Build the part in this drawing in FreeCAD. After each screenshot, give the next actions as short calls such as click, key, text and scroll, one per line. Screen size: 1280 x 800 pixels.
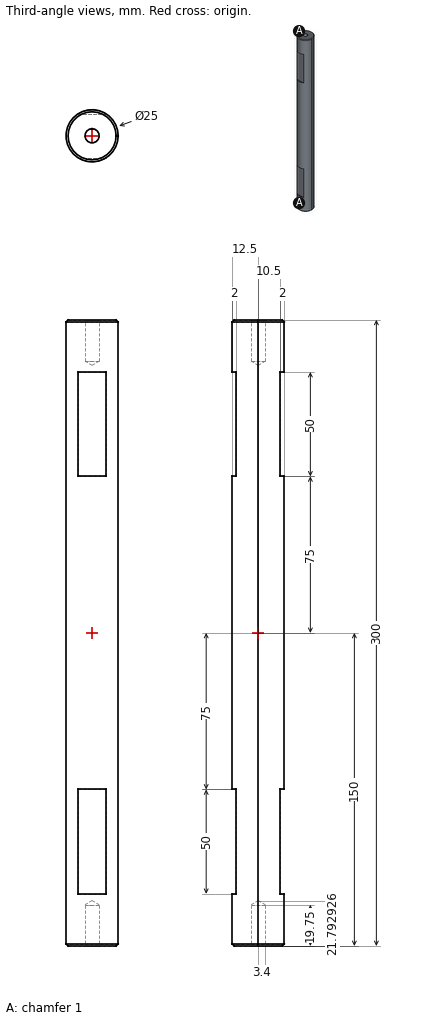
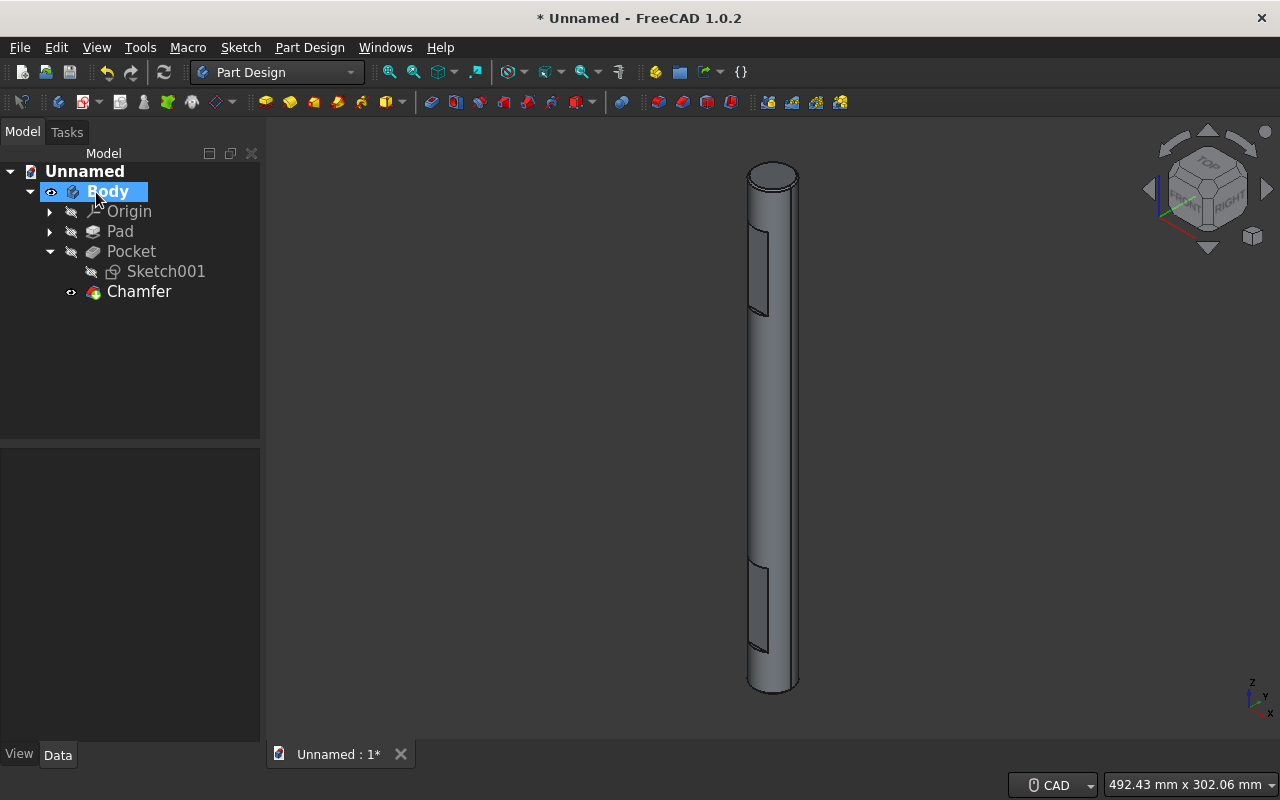
click(84, 102)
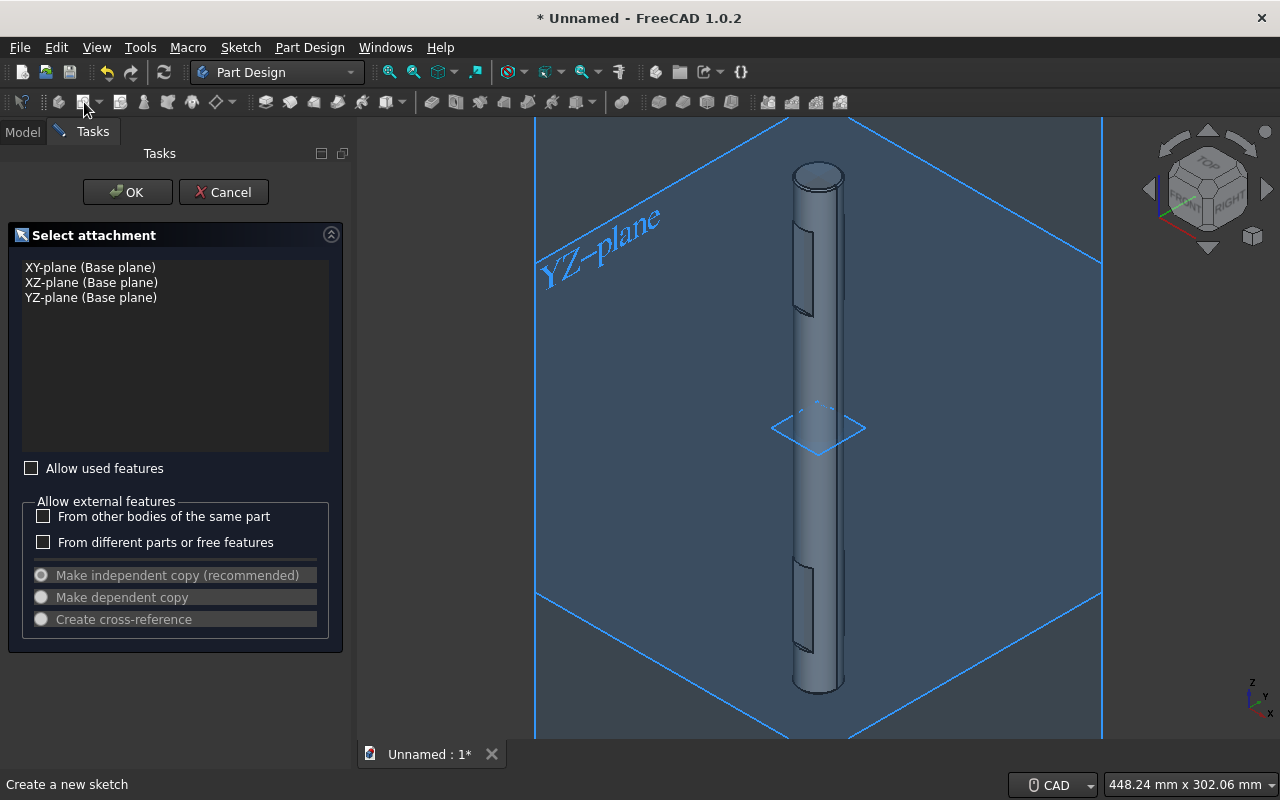
click(82, 298)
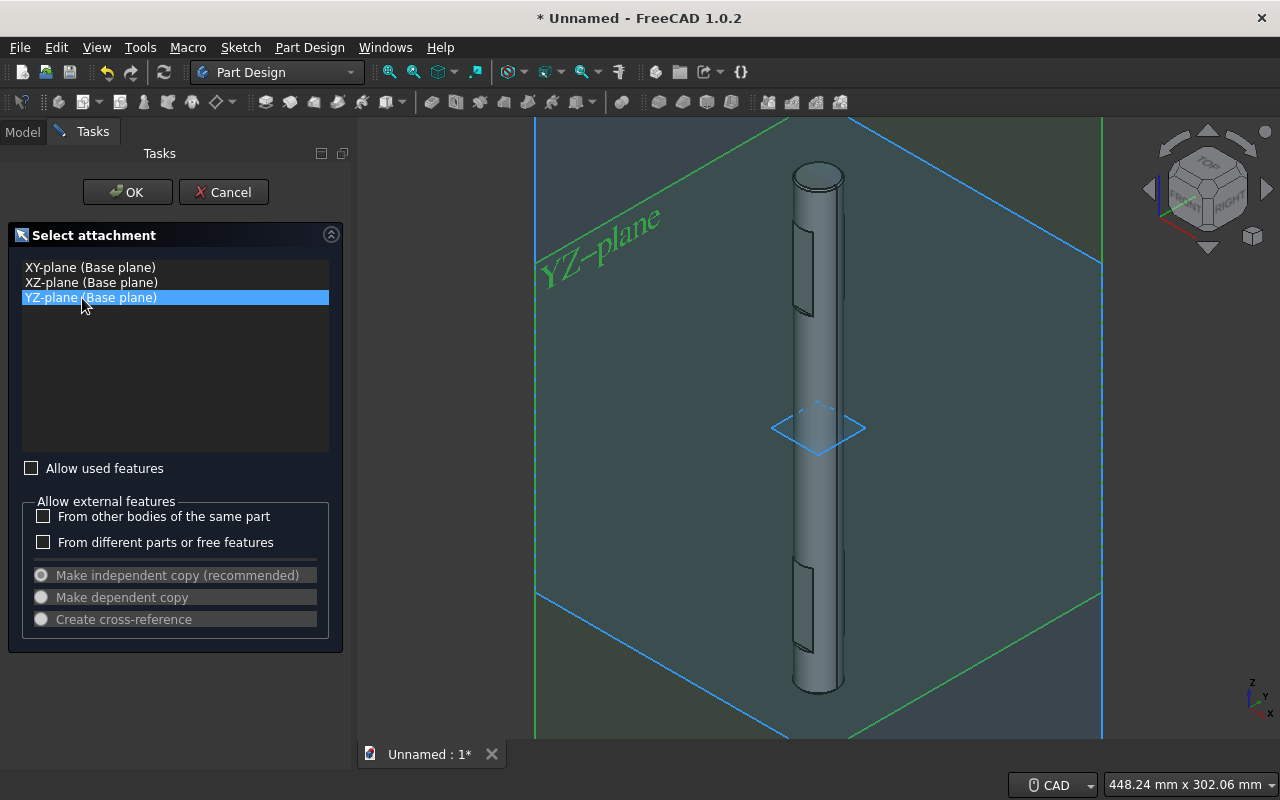
click(128, 192)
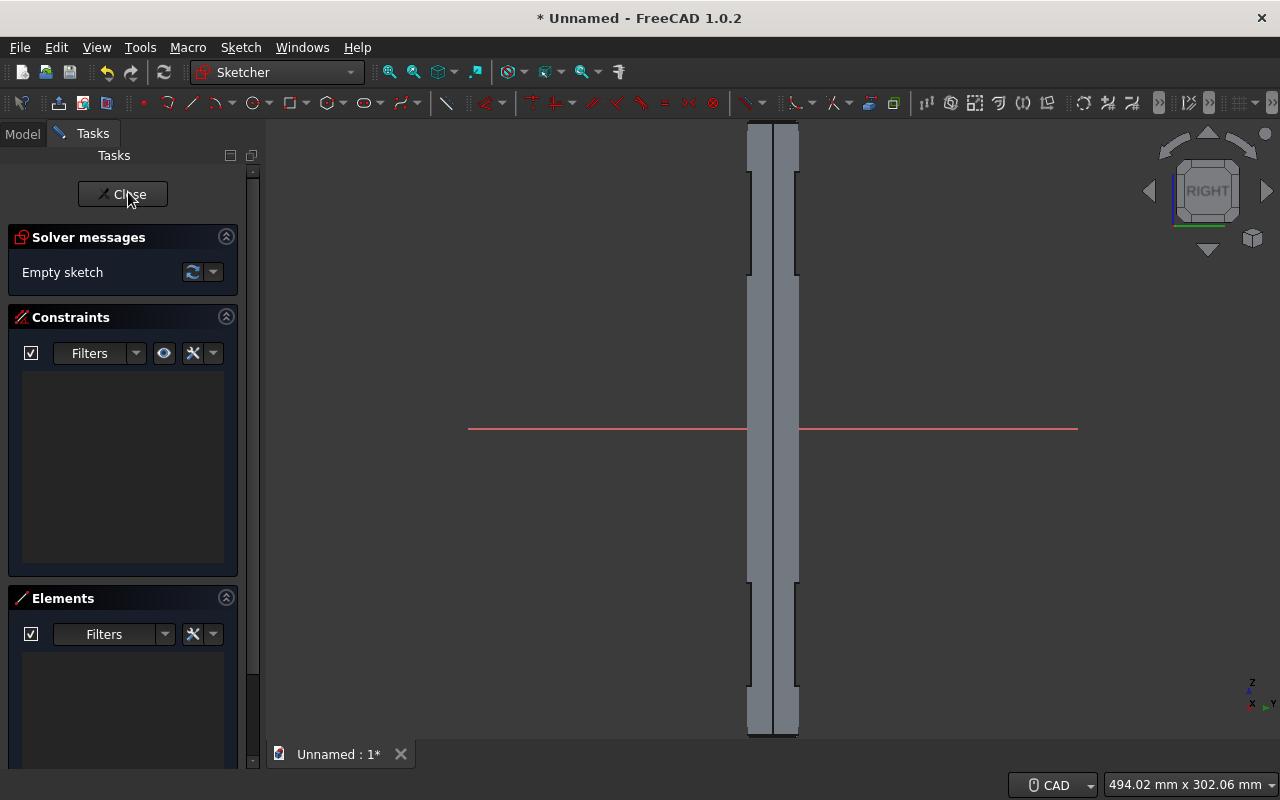
click(108, 104)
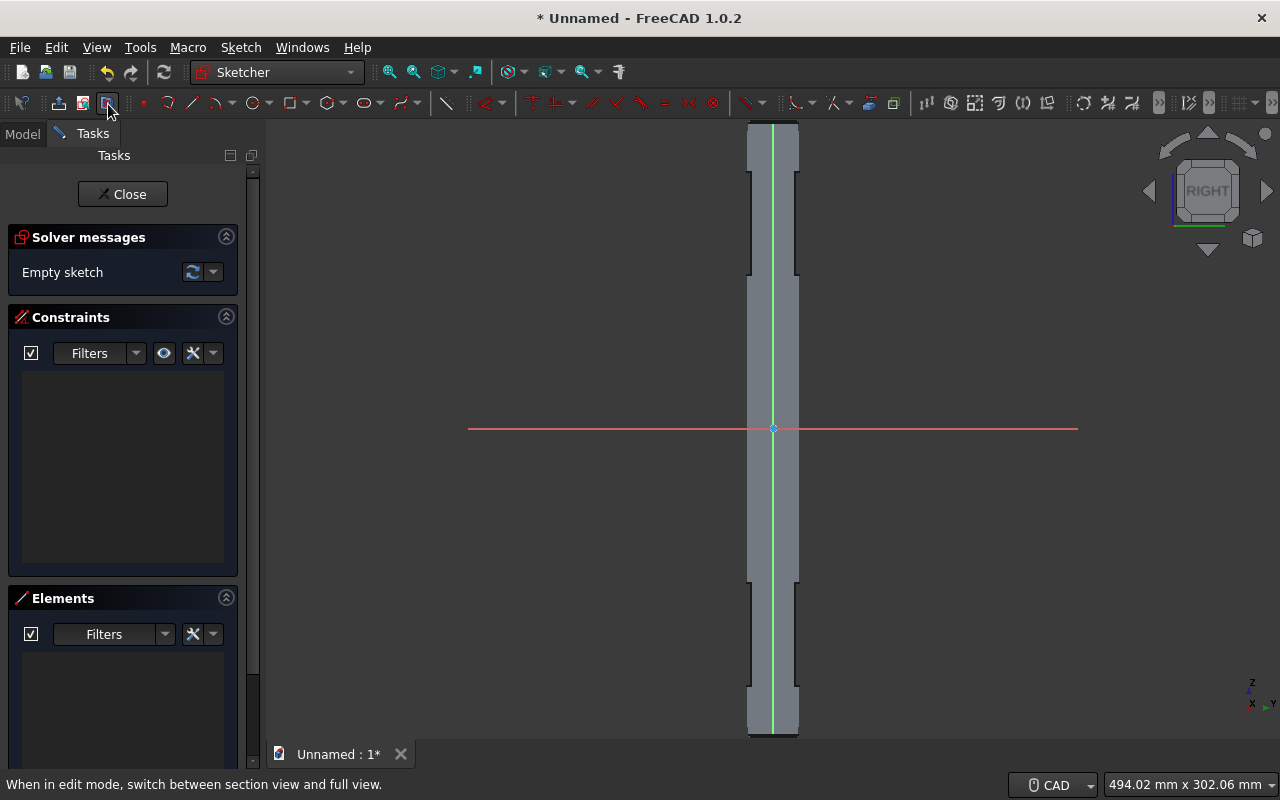
scroll(704, 429, down, 5)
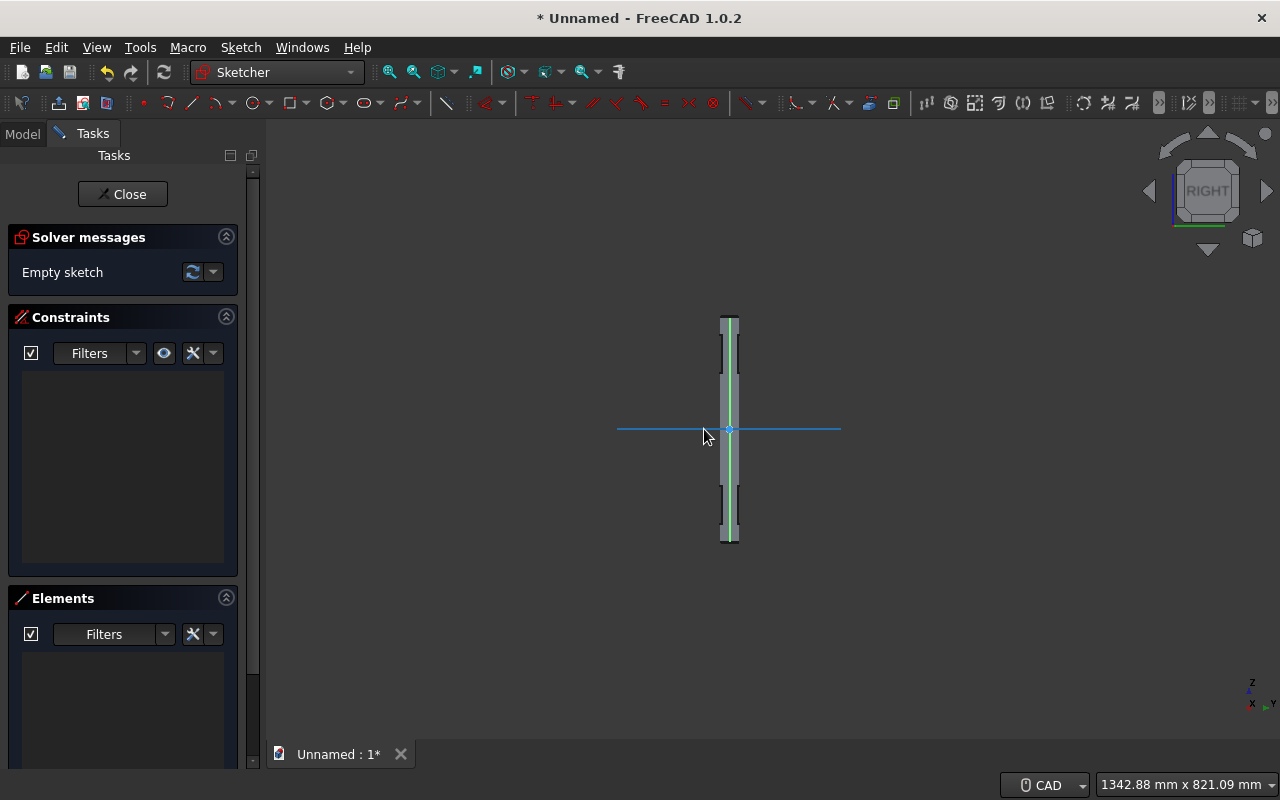
scroll(732, 540, up, 15)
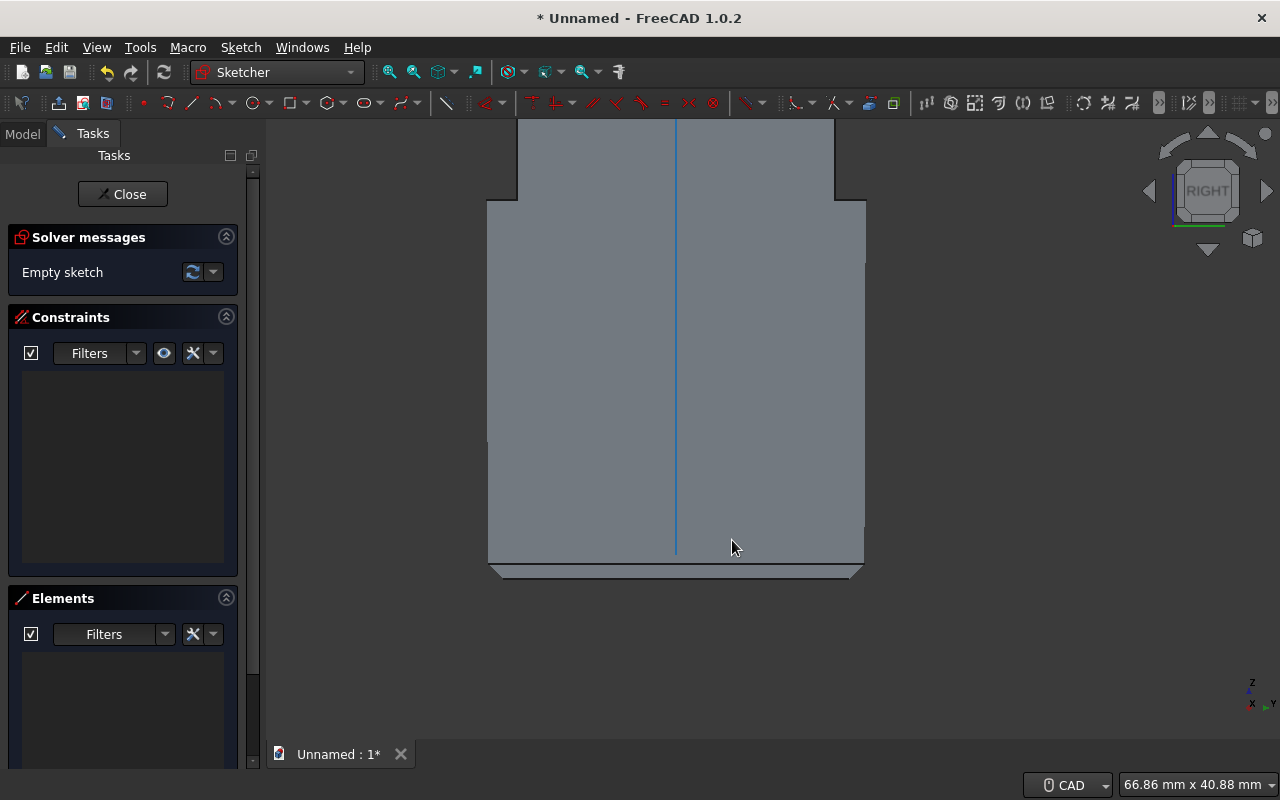
click(168, 104)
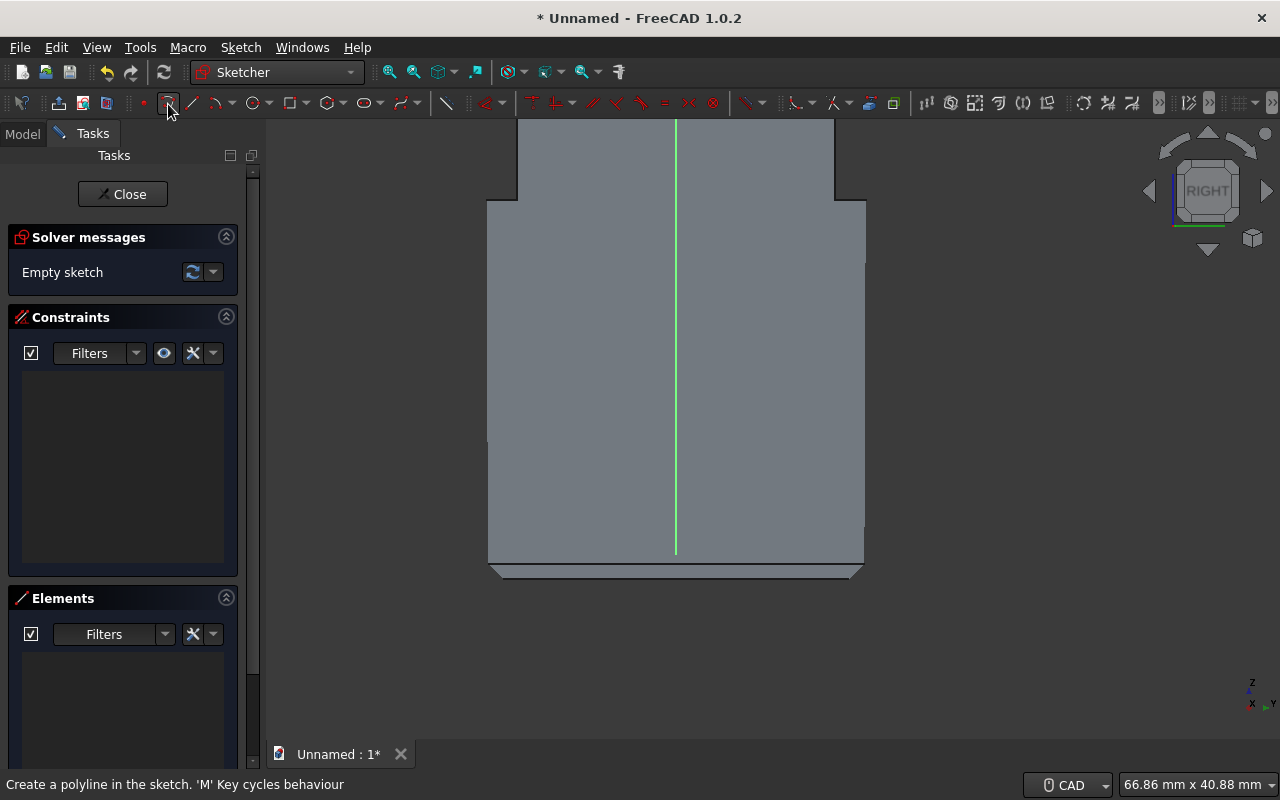
click(676, 248)
click(685, 579)
click(728, 579)
click(728, 279)
click(676, 249)
key(Escape)
key(Escape)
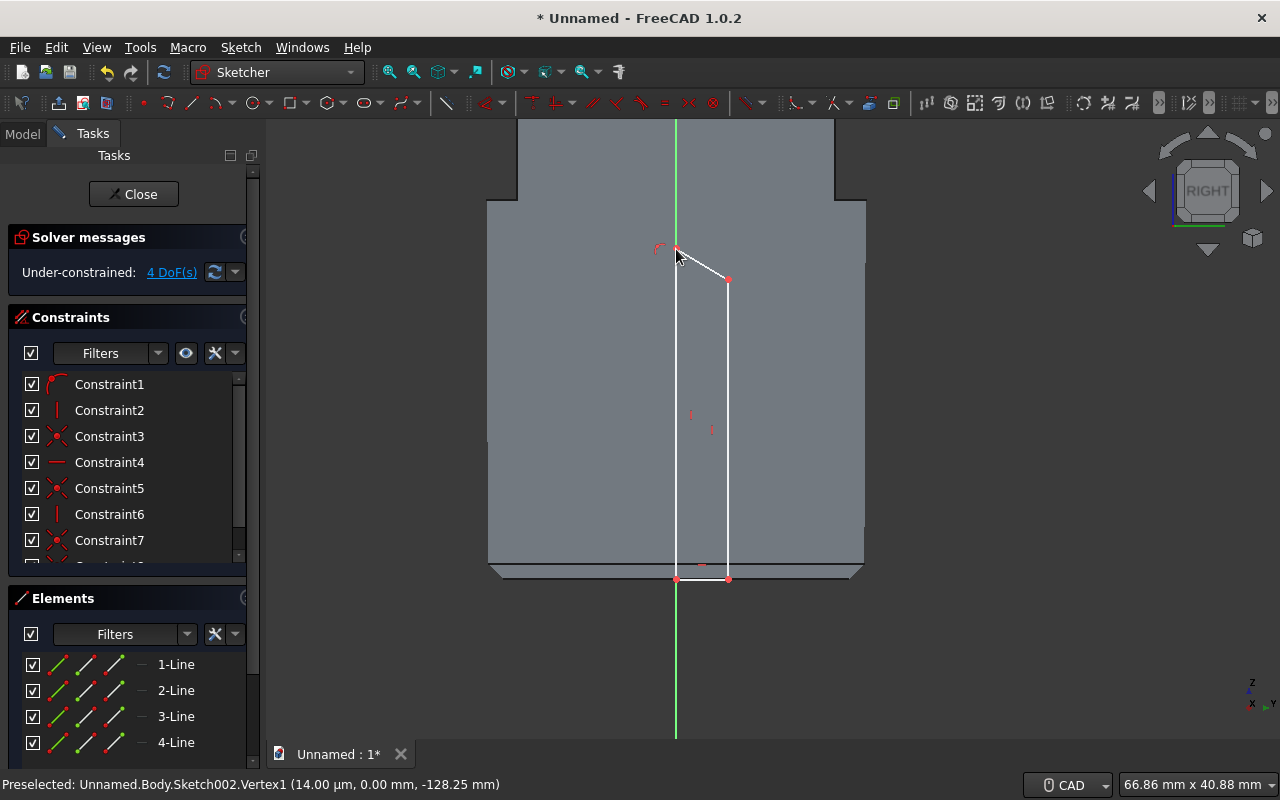
click(486, 104)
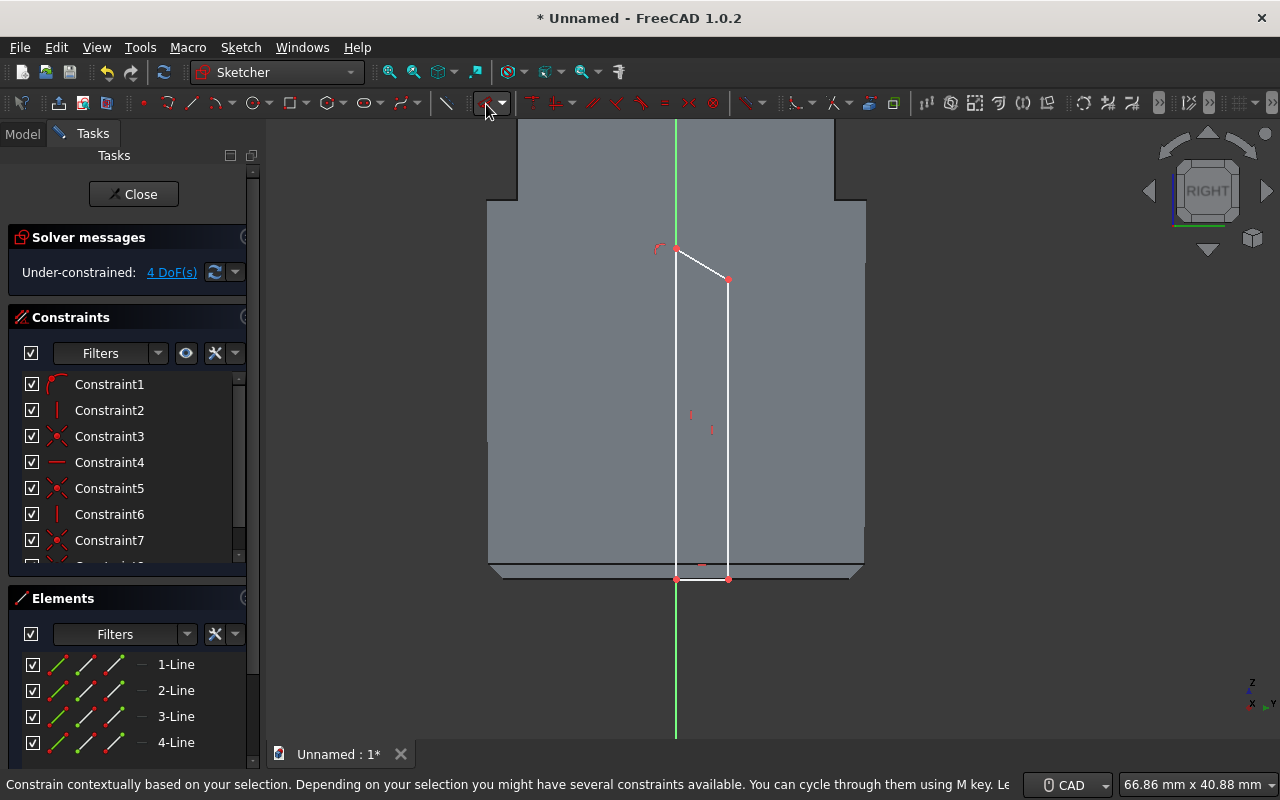
click(692, 580)
click(702, 614)